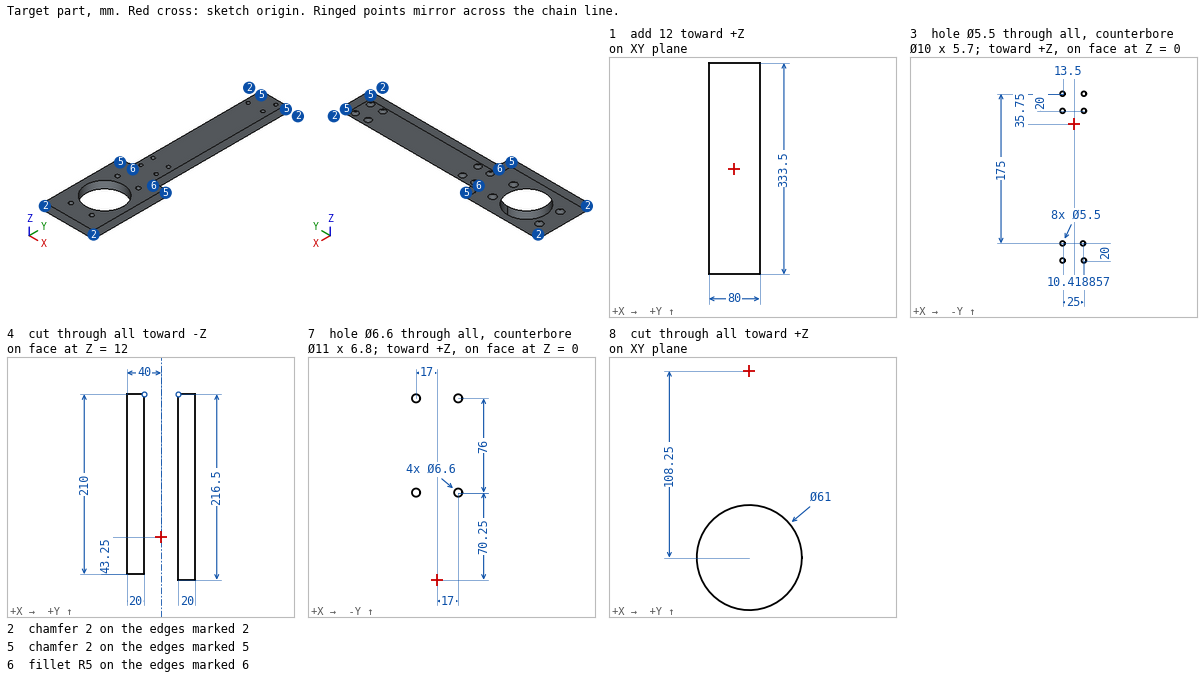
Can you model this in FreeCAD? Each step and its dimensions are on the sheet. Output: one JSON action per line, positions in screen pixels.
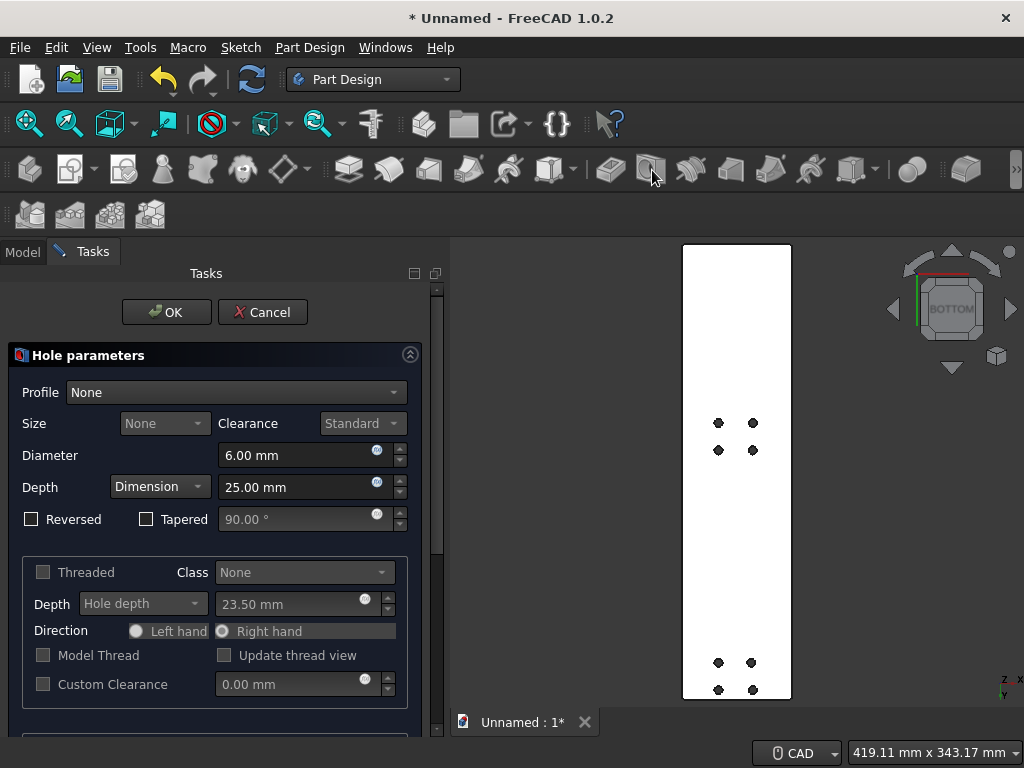
{"action": "triple_click", "coordinate": [305, 455]}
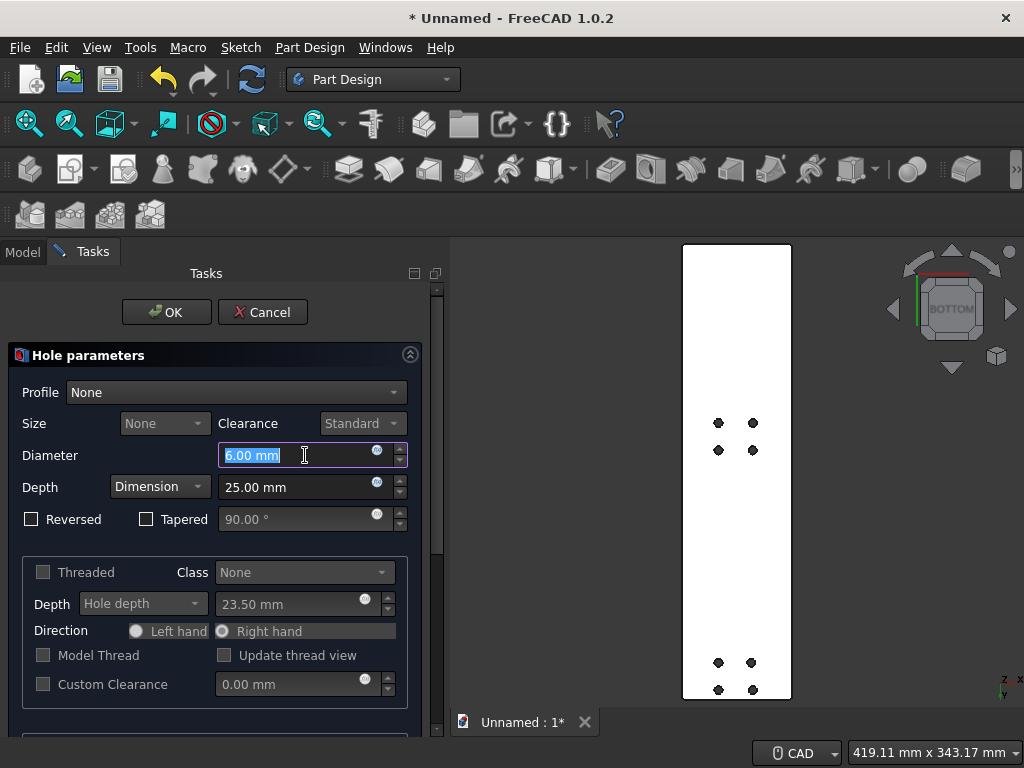
{"action": "type", "text": "5.5"}
{"action": "key", "text": "Tab"}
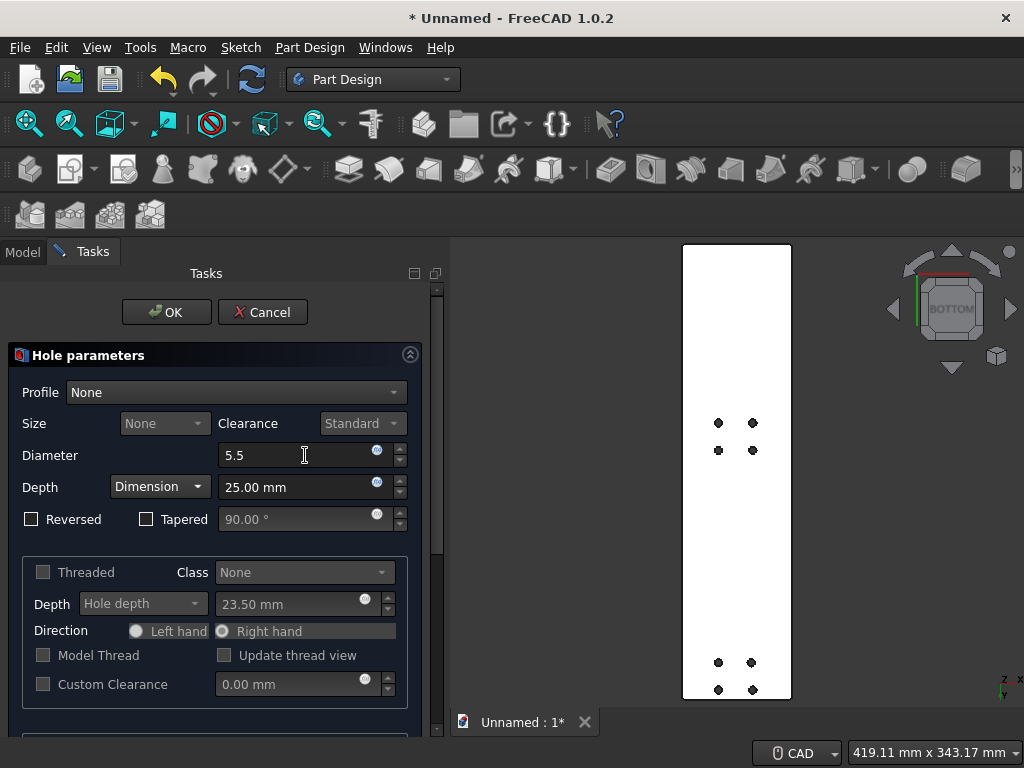
{"action": "left_click", "coordinate": [161, 486]}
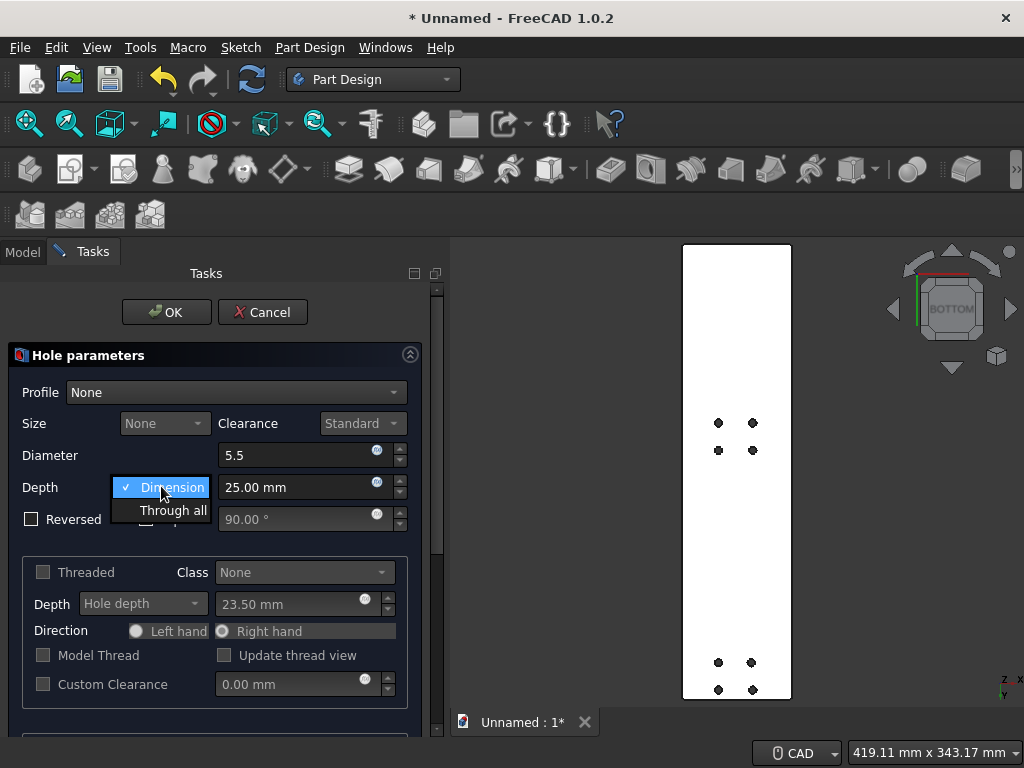
{"action": "left_click", "coordinate": [160, 510]}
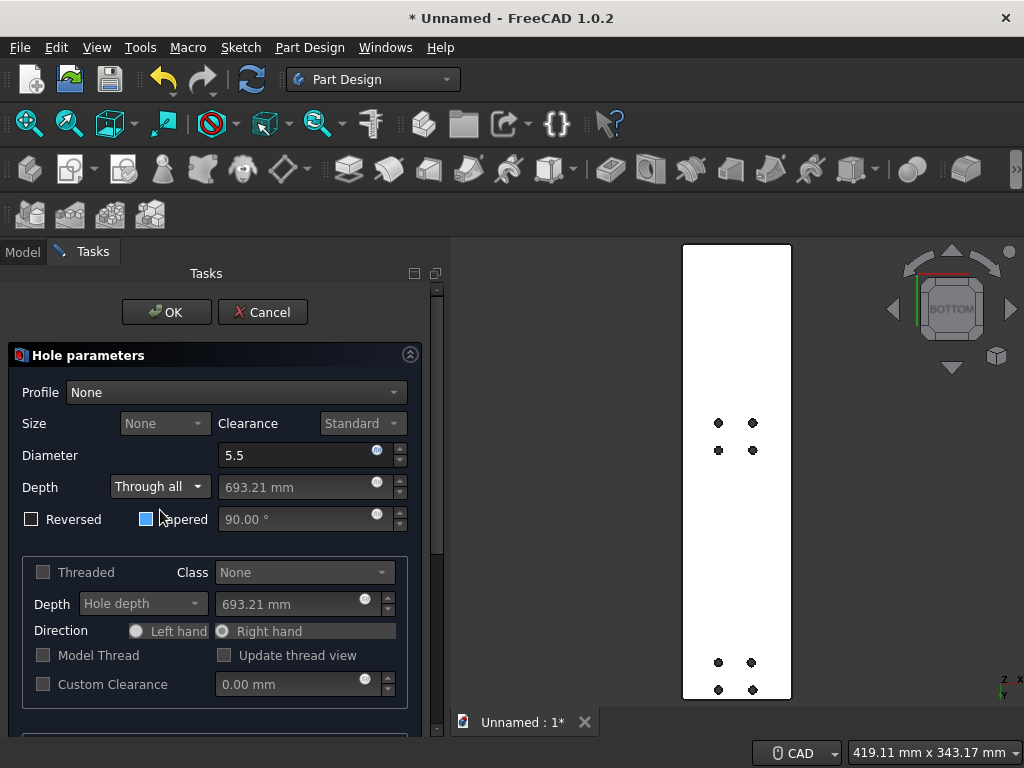
{"action": "scroll", "coordinate": [437, 510], "scroll_direction": "down", "scroll_amount": 2}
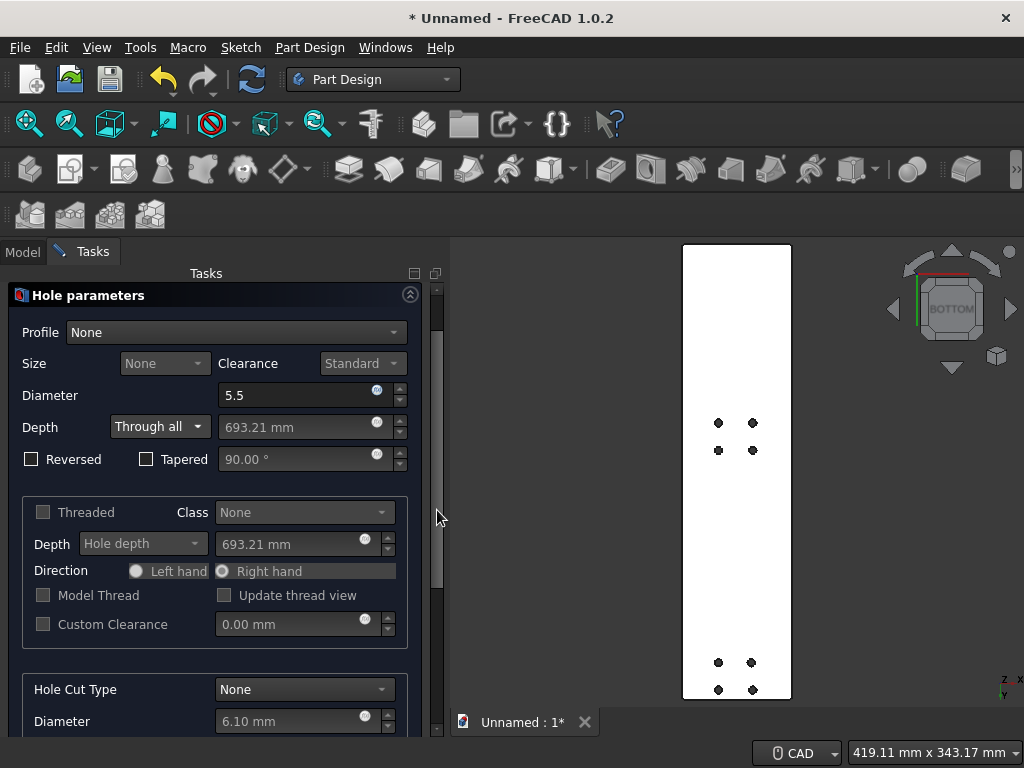
{"action": "left_click", "coordinate": [306, 630]}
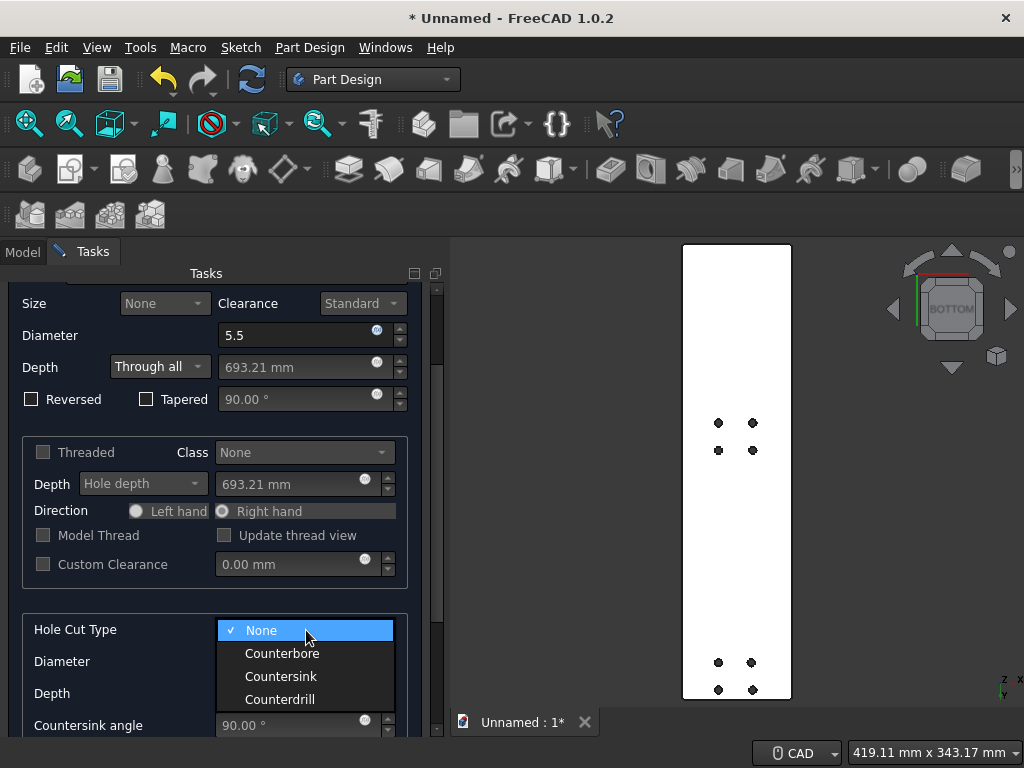
{"action": "left_click", "coordinate": [304, 654]}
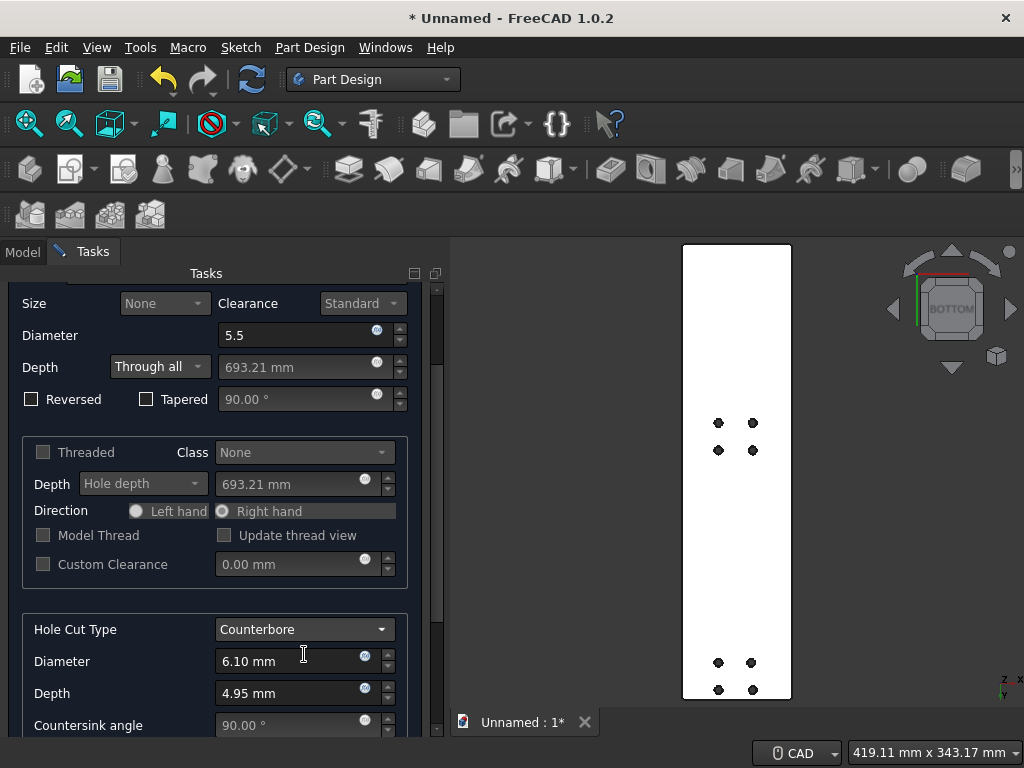
{"action": "triple_click", "coordinate": [298, 661]}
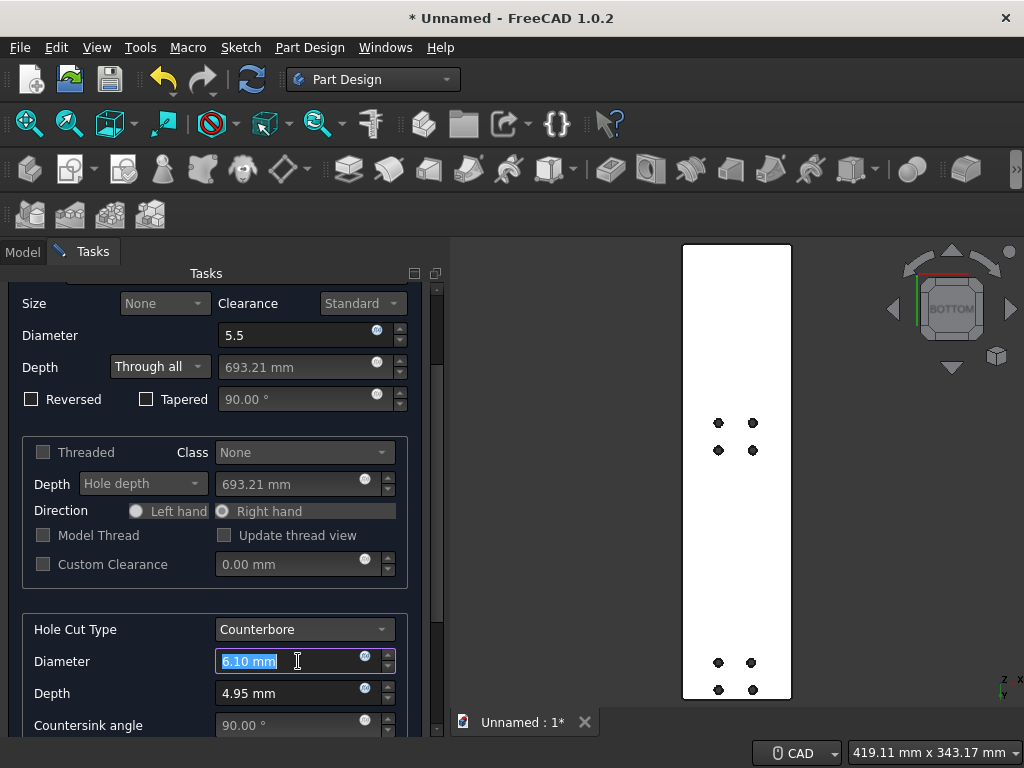
{"action": "type", "text": "10"}
{"action": "key", "text": "Tab"}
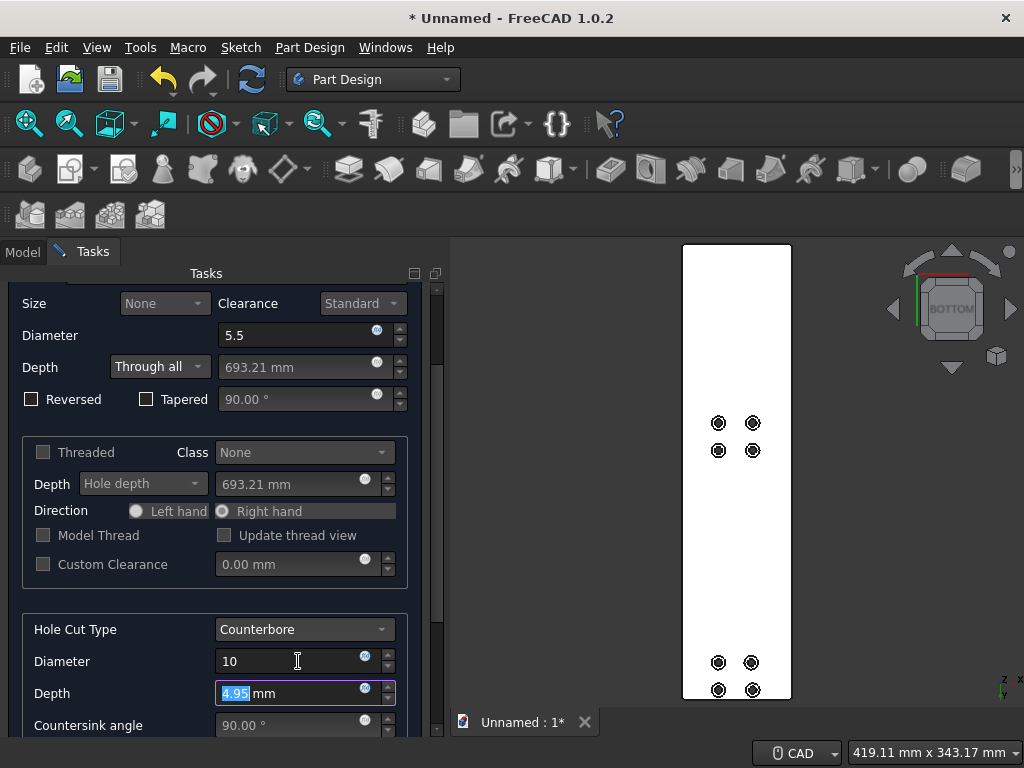
{"action": "type", "text": "5.7"}
{"action": "key", "text": "Tab"}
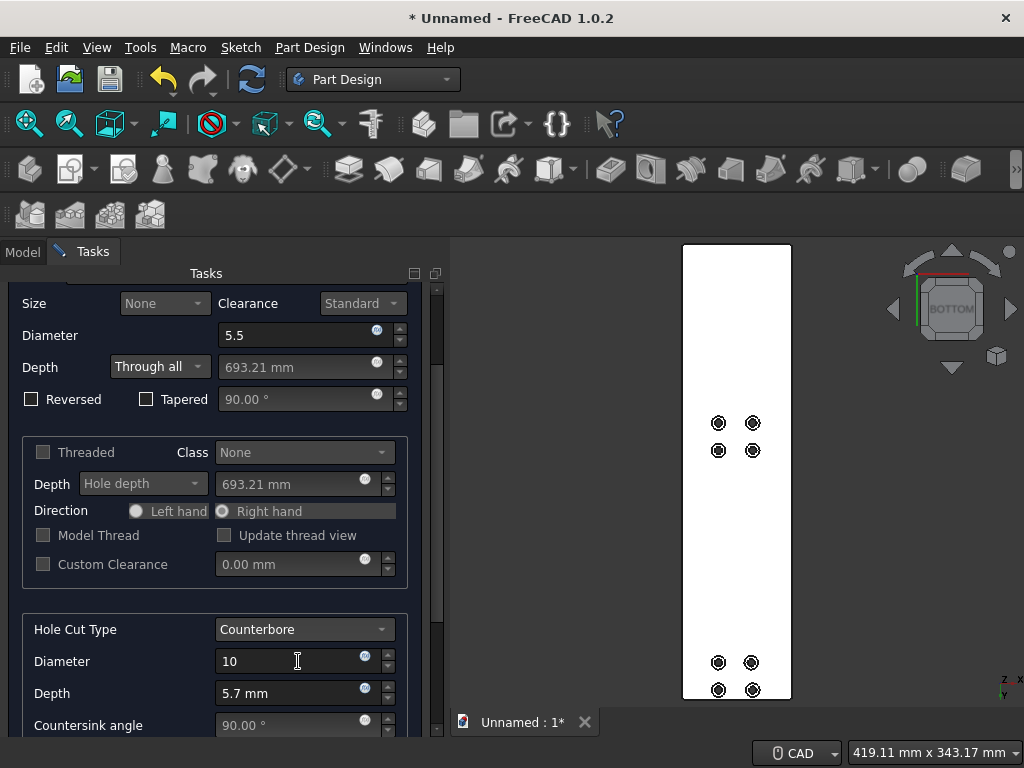
{"action": "scroll", "coordinate": [437, 510], "scroll_direction": "up", "scroll_amount": 3}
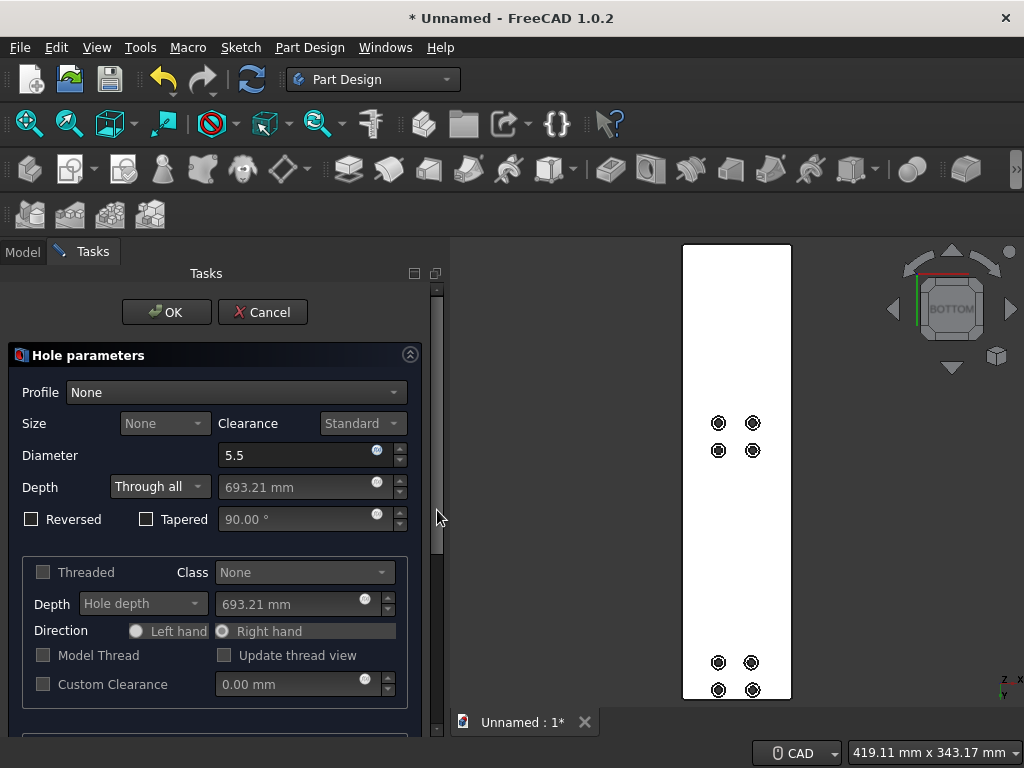
{"action": "left_click", "coordinate": [167, 312]}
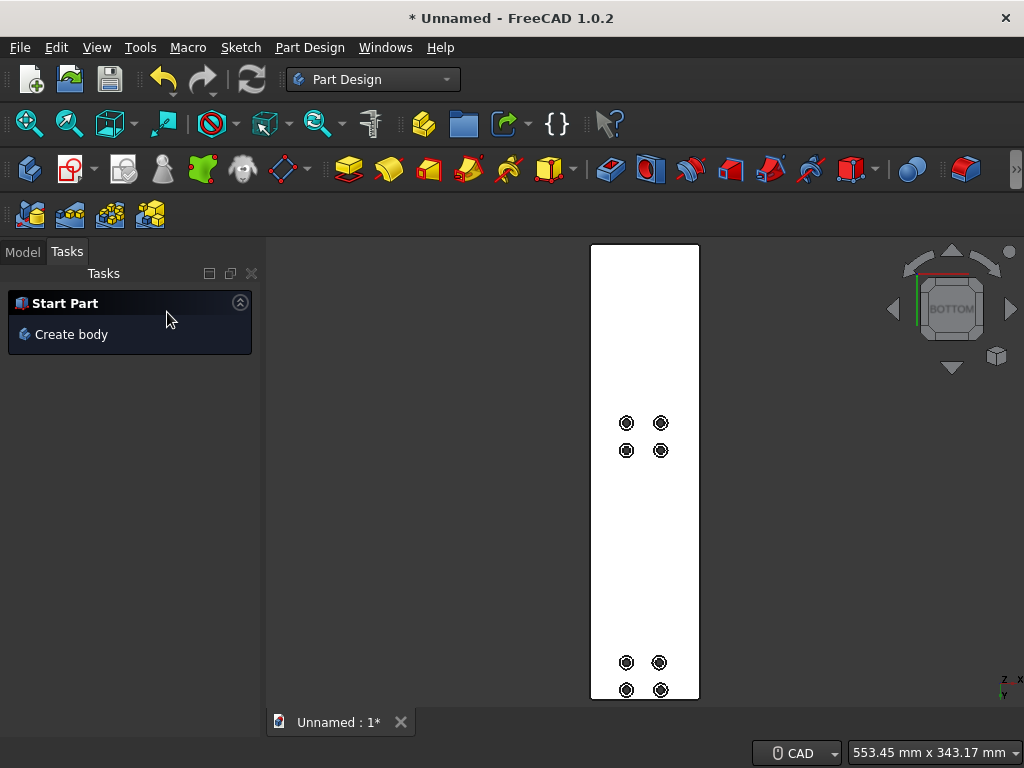
{"action": "key", "text": "0"}